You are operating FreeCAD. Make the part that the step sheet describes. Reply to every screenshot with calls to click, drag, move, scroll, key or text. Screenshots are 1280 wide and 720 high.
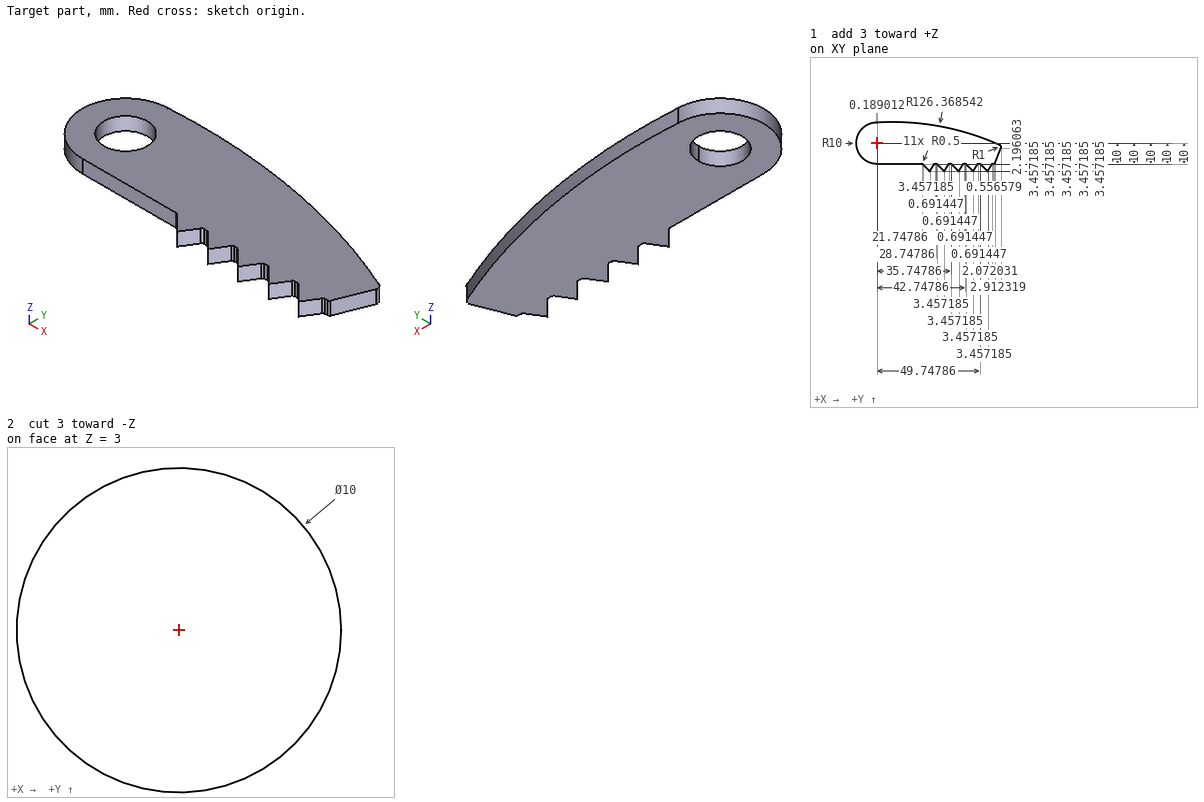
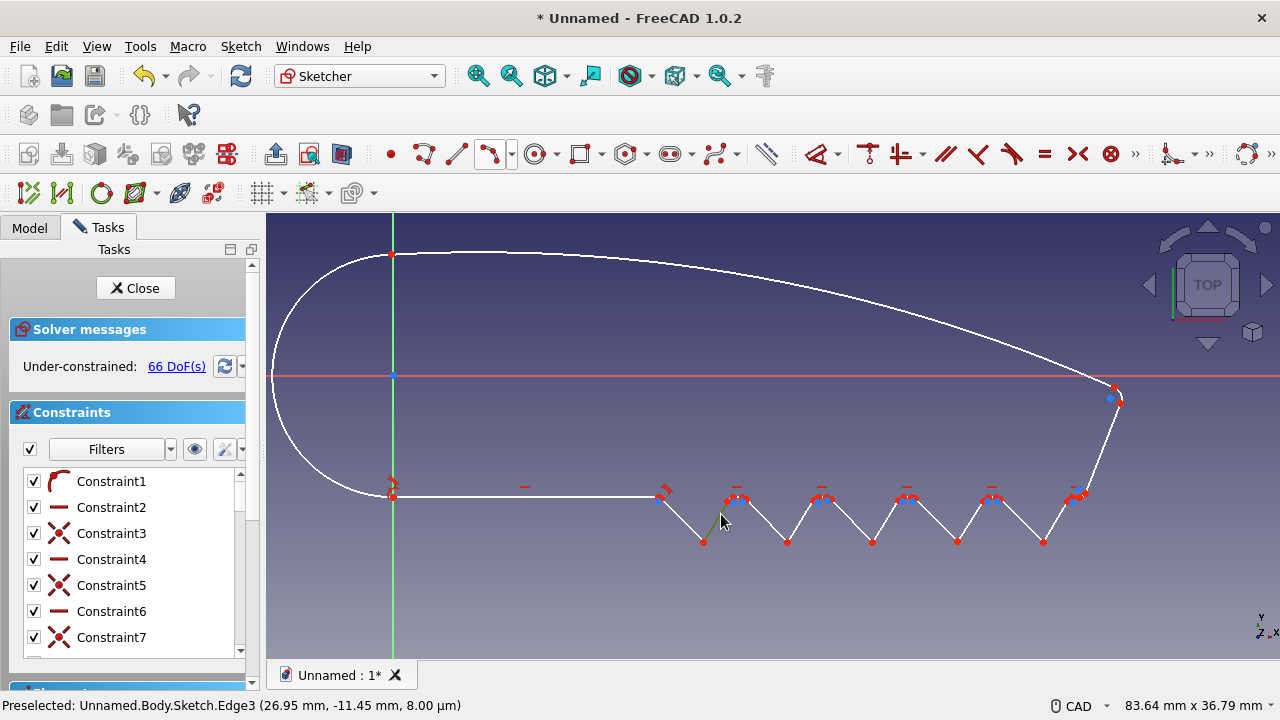
scroll(730, 498, up, 7)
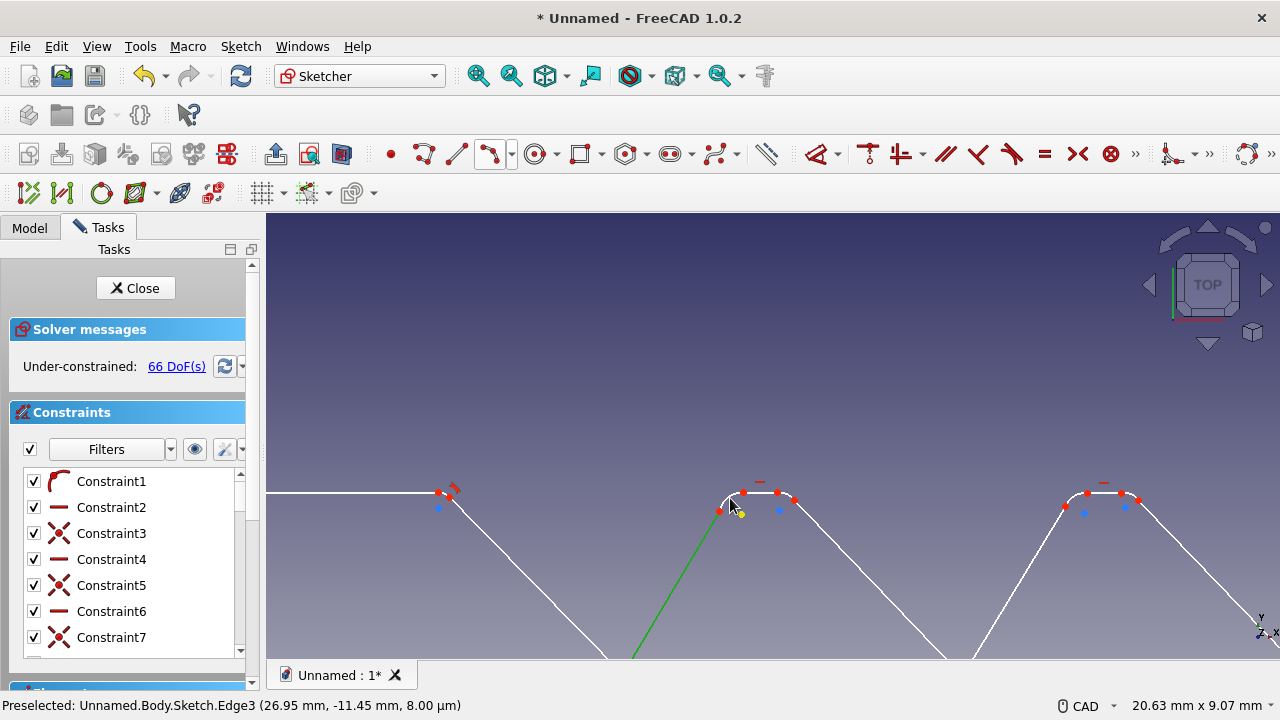
click(728, 497)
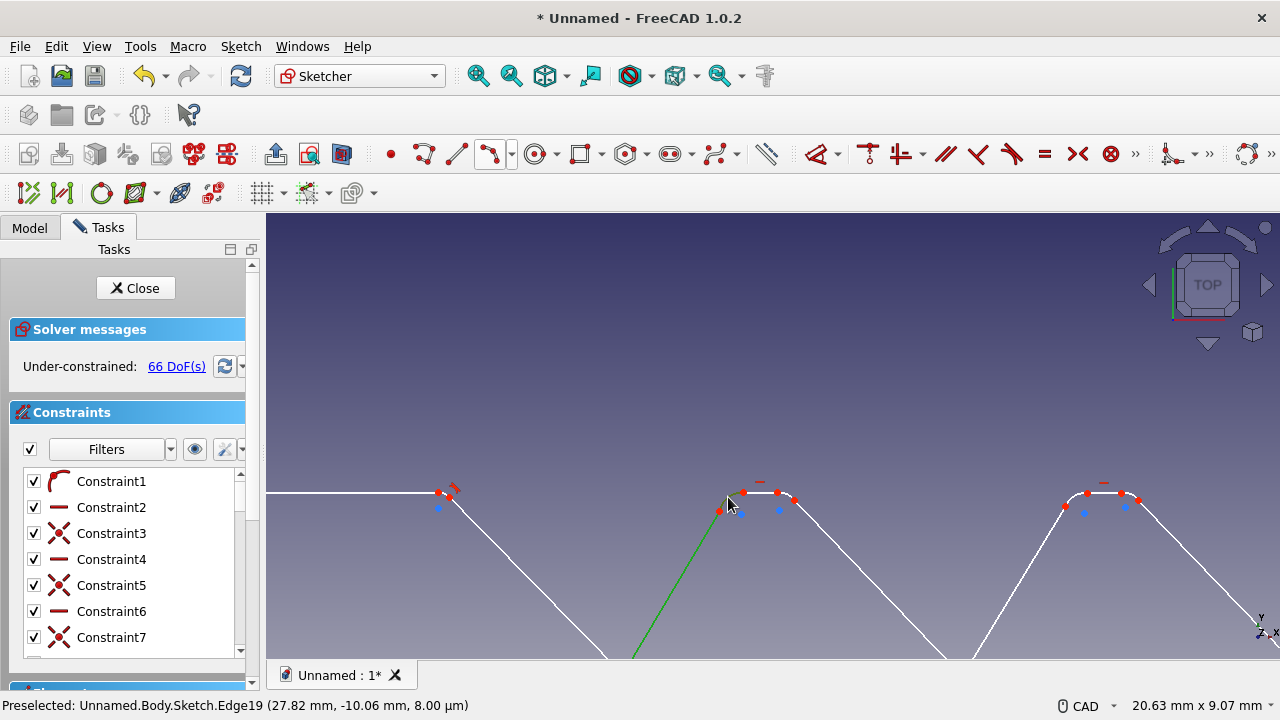
key(t)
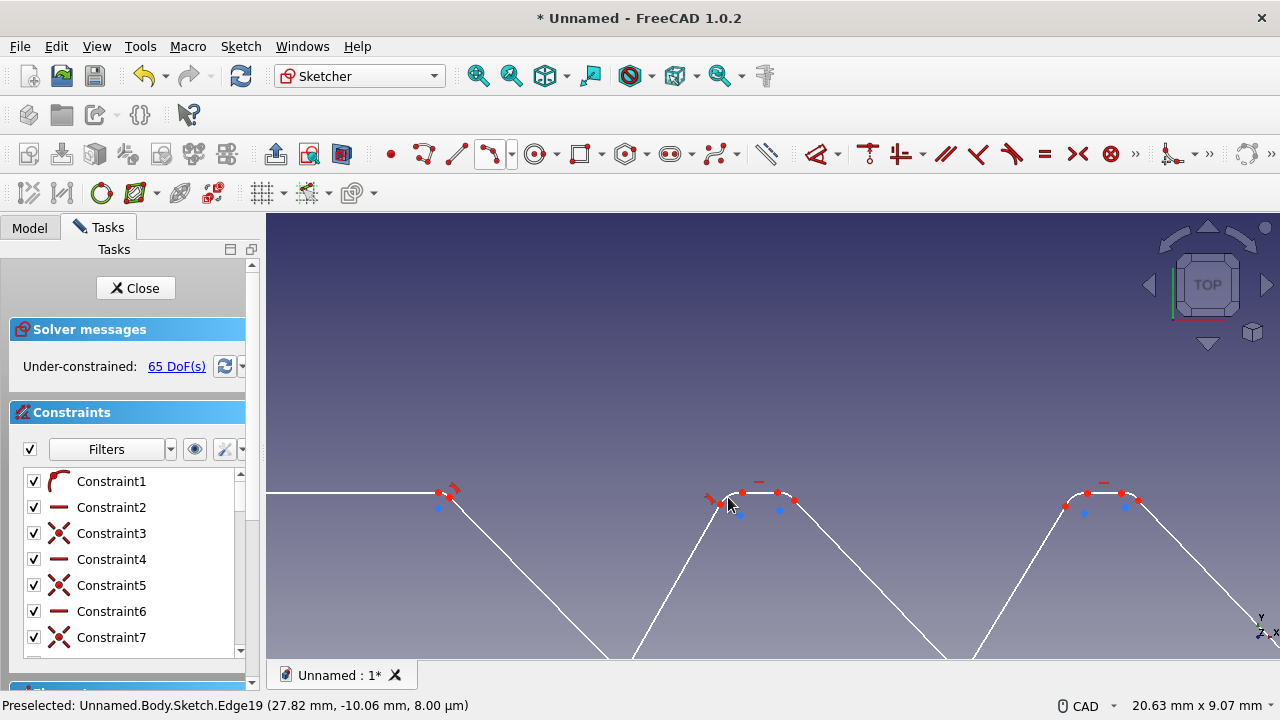
scroll(753, 493, up, 2)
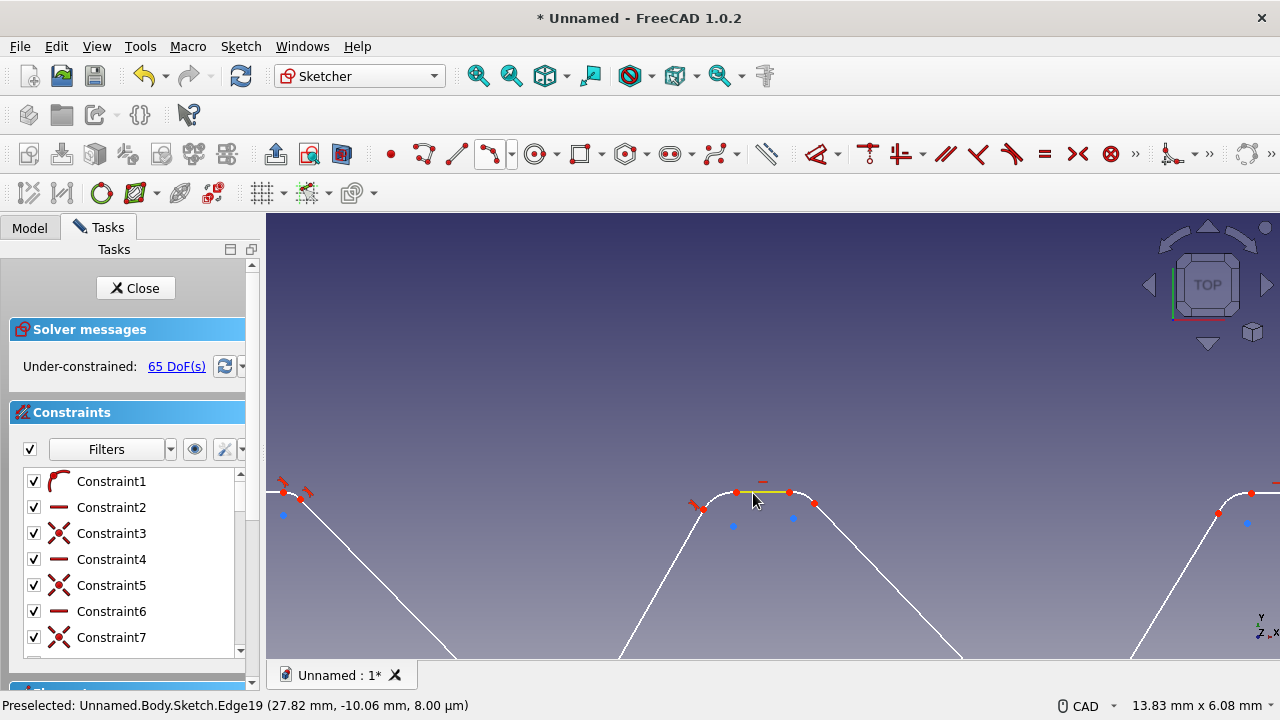
click(752, 492)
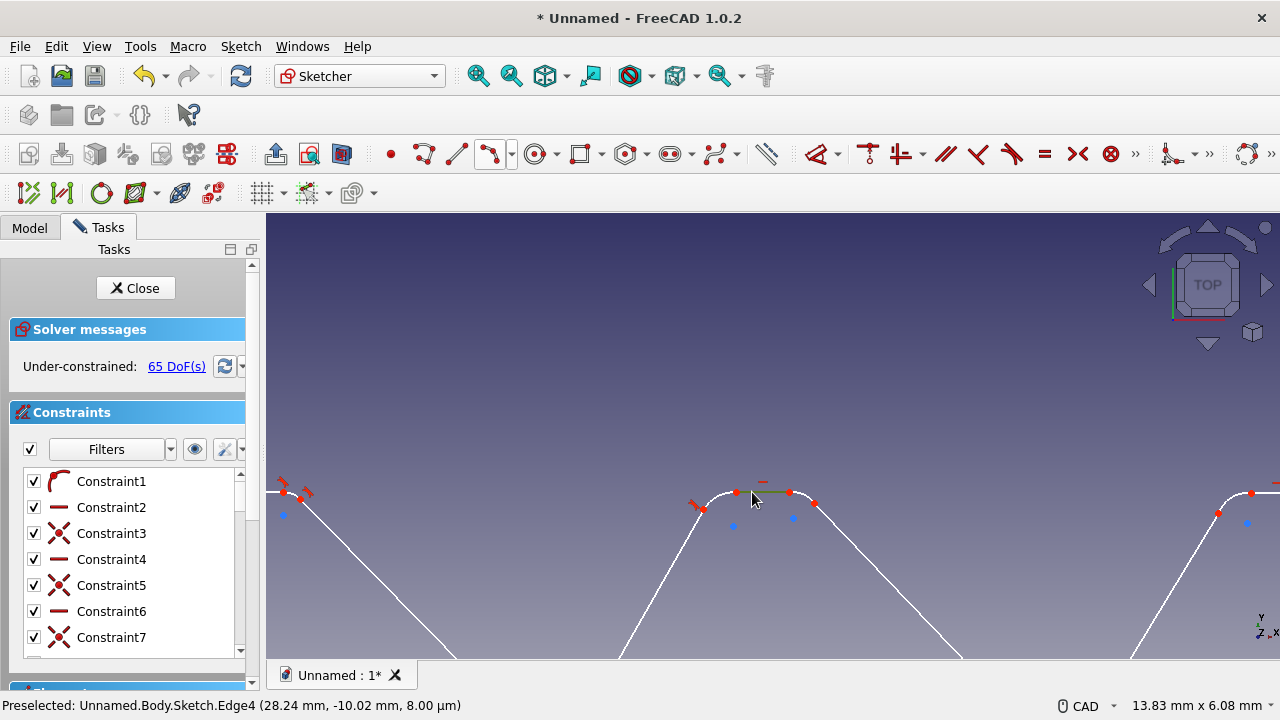
click(725, 493)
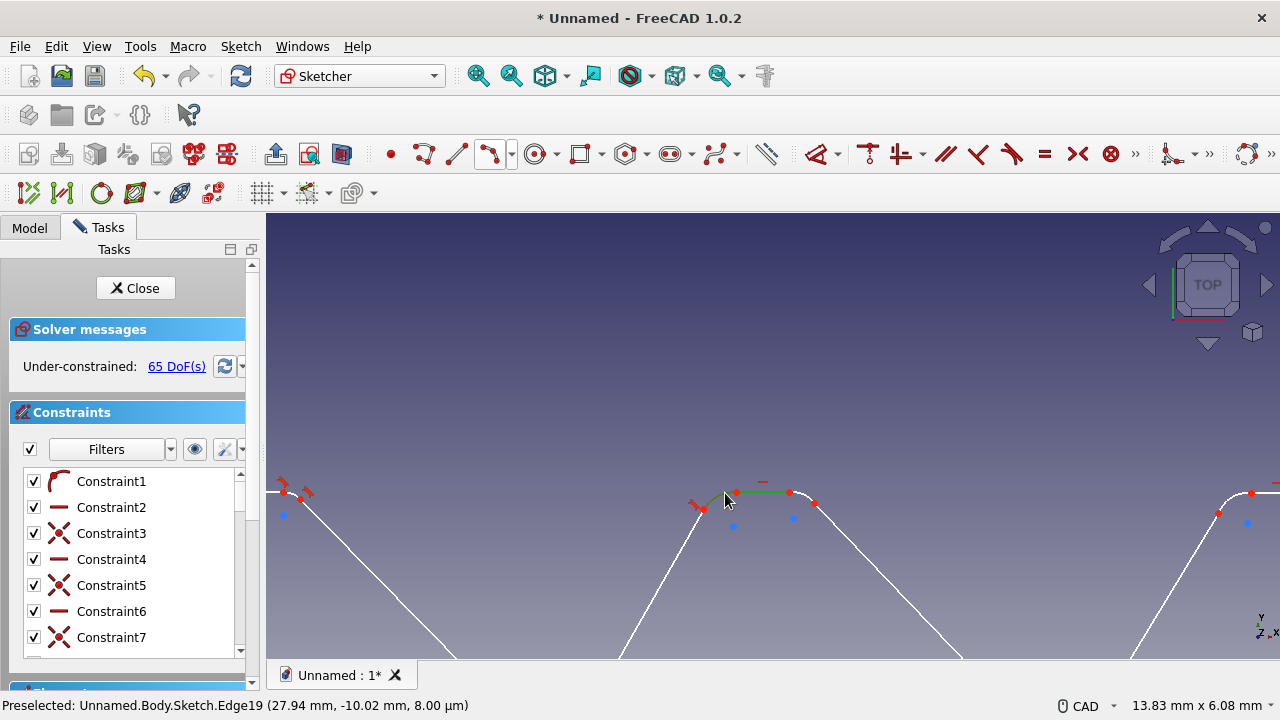
click(1012, 154)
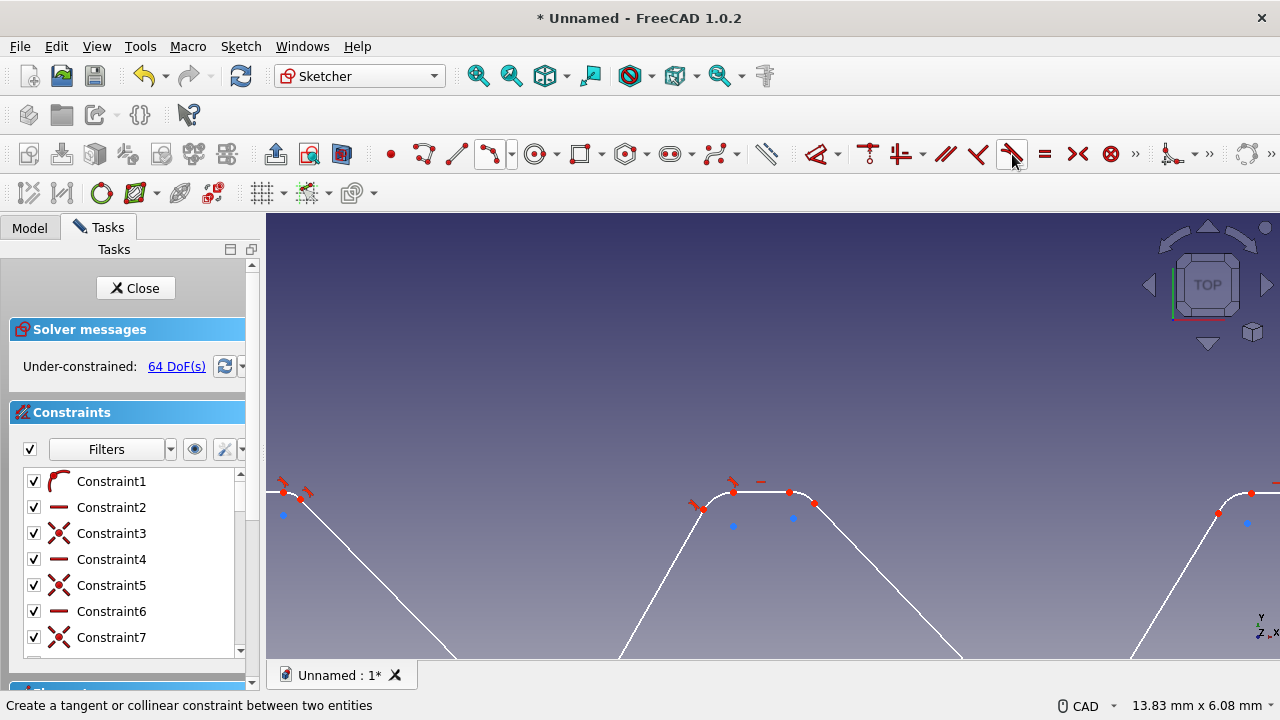
click(750, 492)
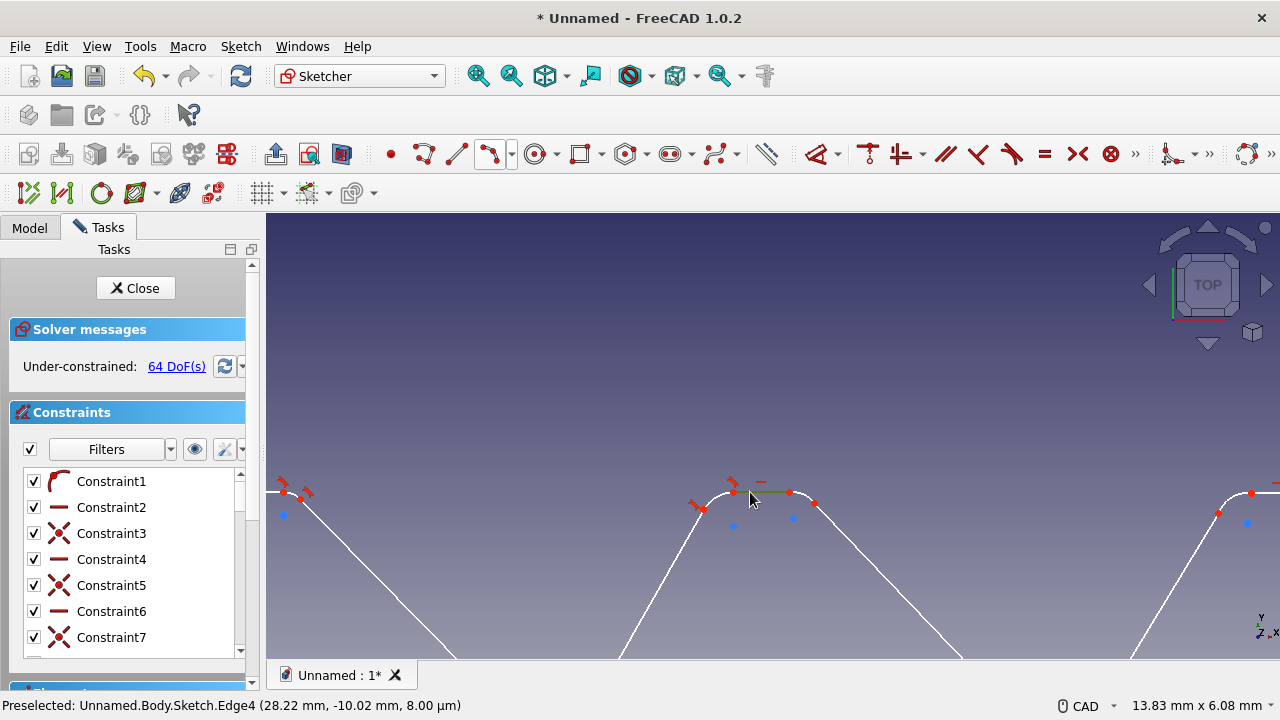
click(803, 494)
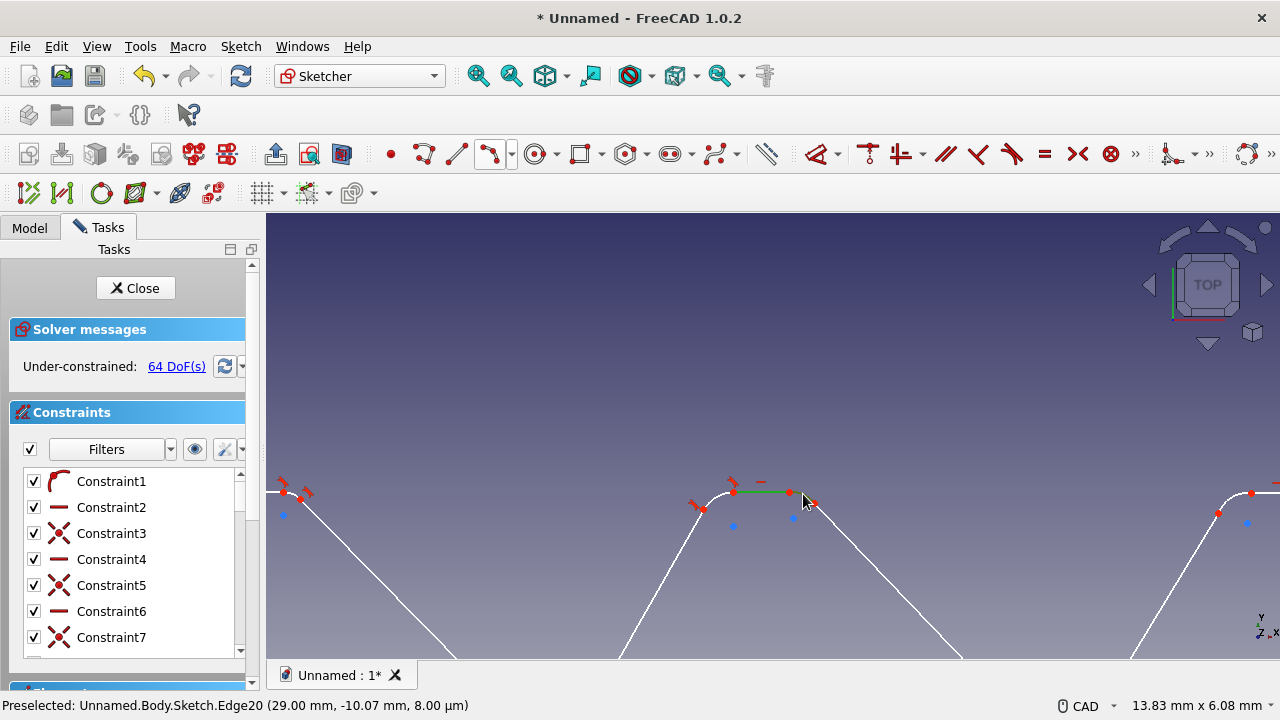
key(t)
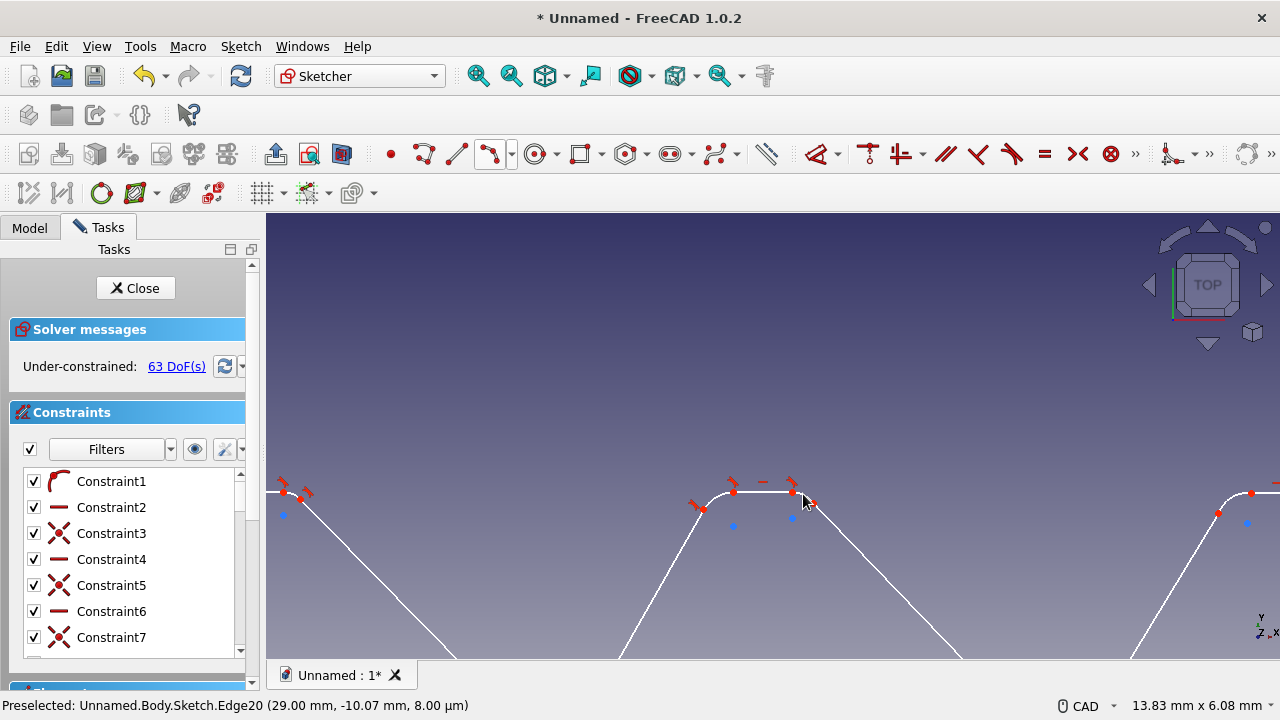
scroll(728, 504, down, 11)